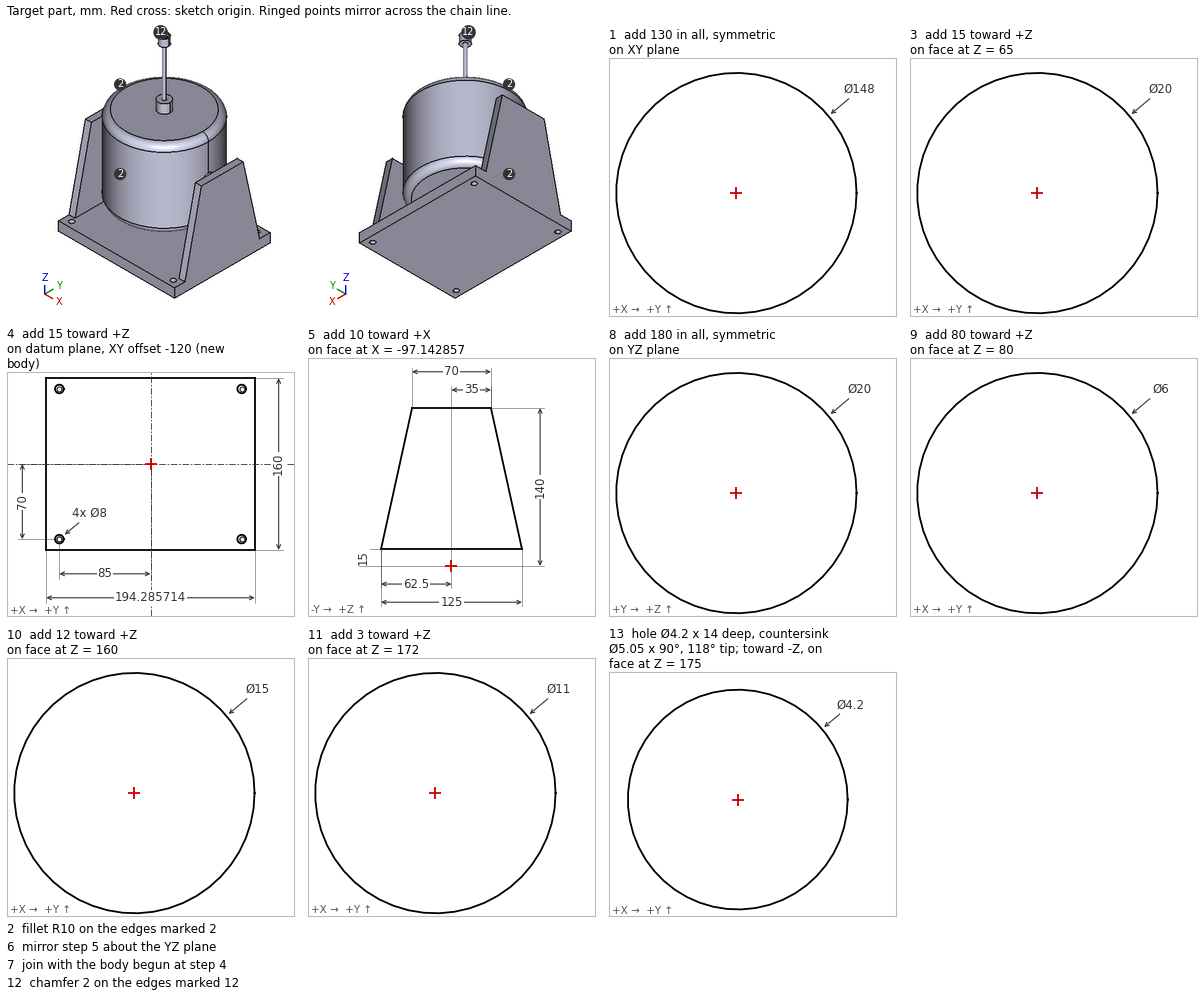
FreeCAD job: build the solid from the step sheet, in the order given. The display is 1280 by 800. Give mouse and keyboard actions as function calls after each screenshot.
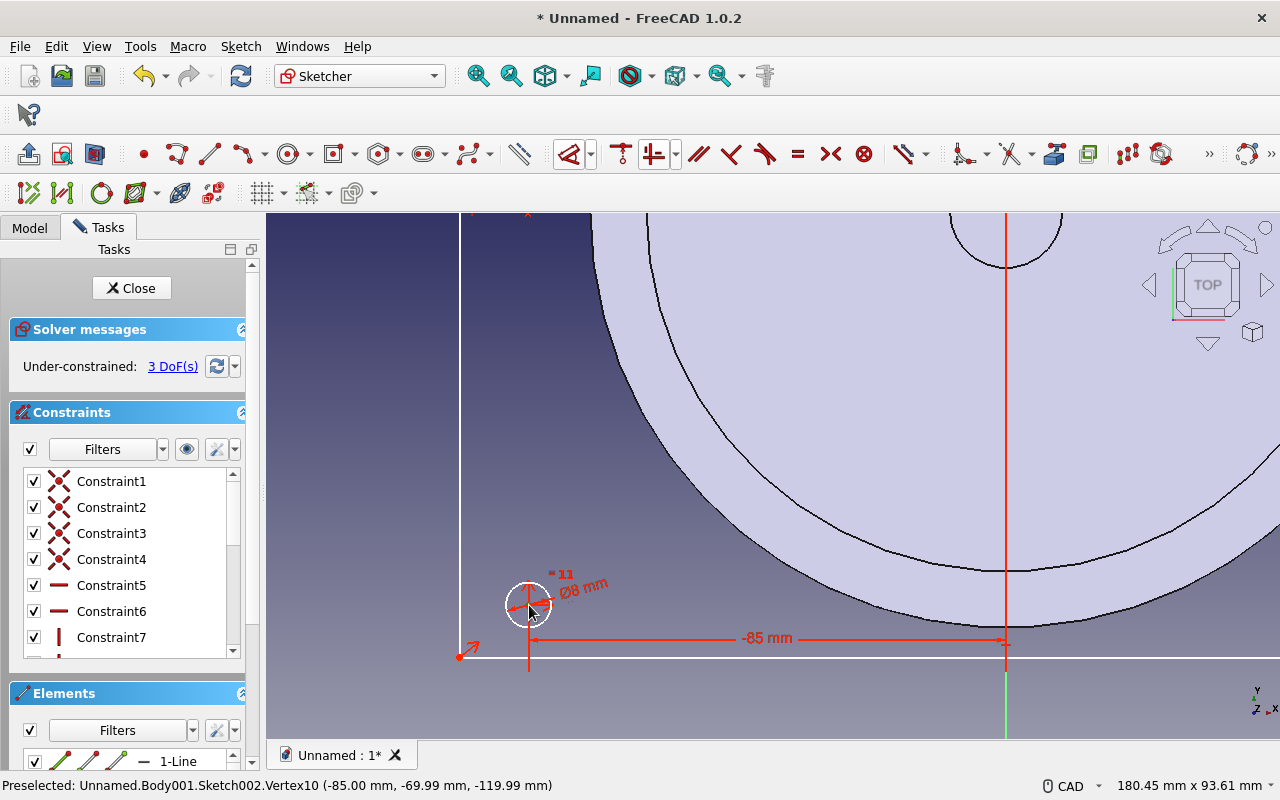
key(i)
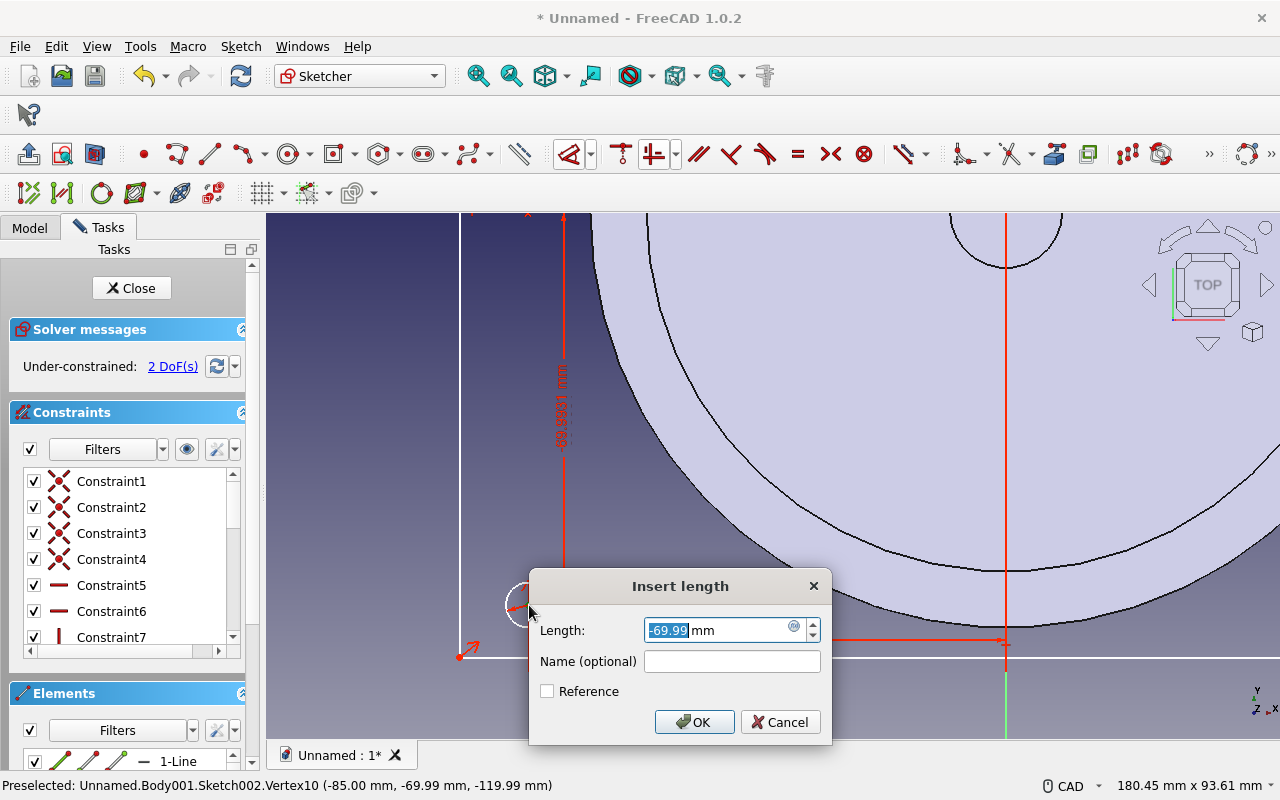
text(-70)
key(Return)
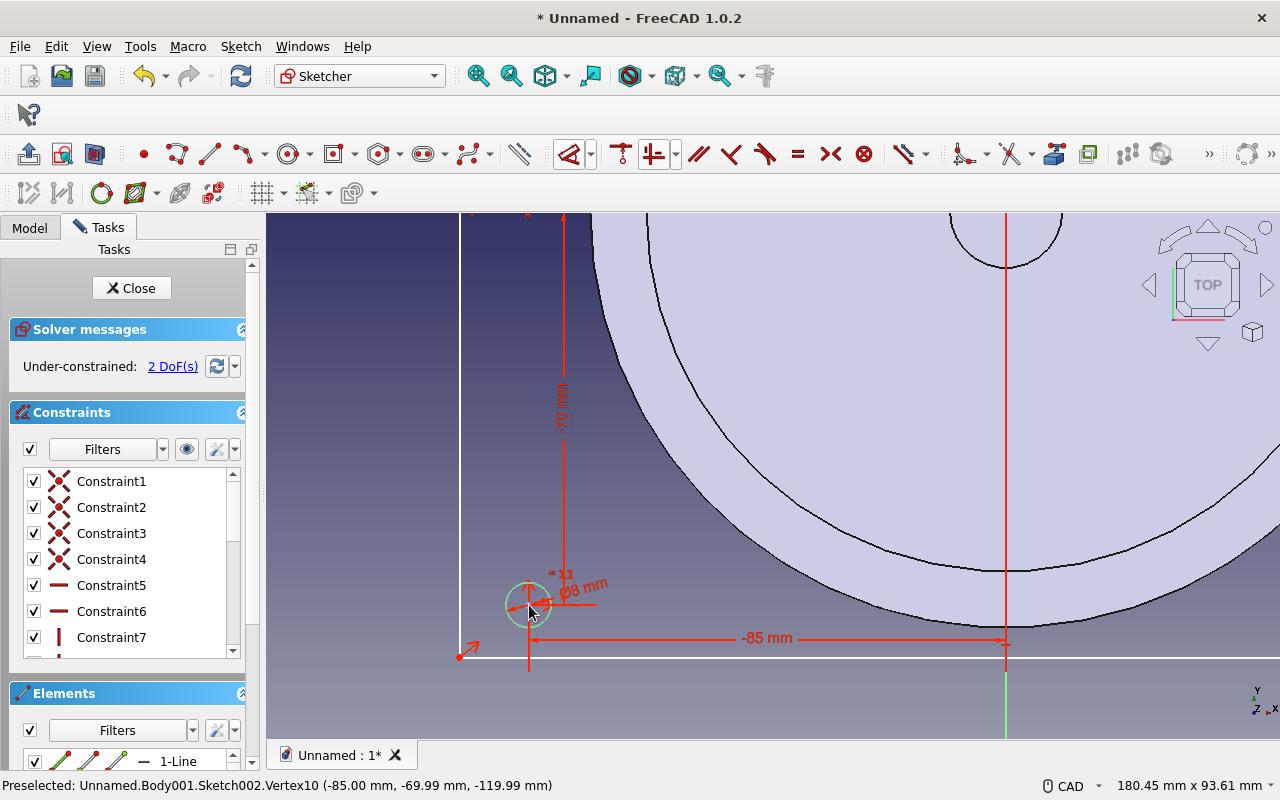
scroll(529, 630, down, 5)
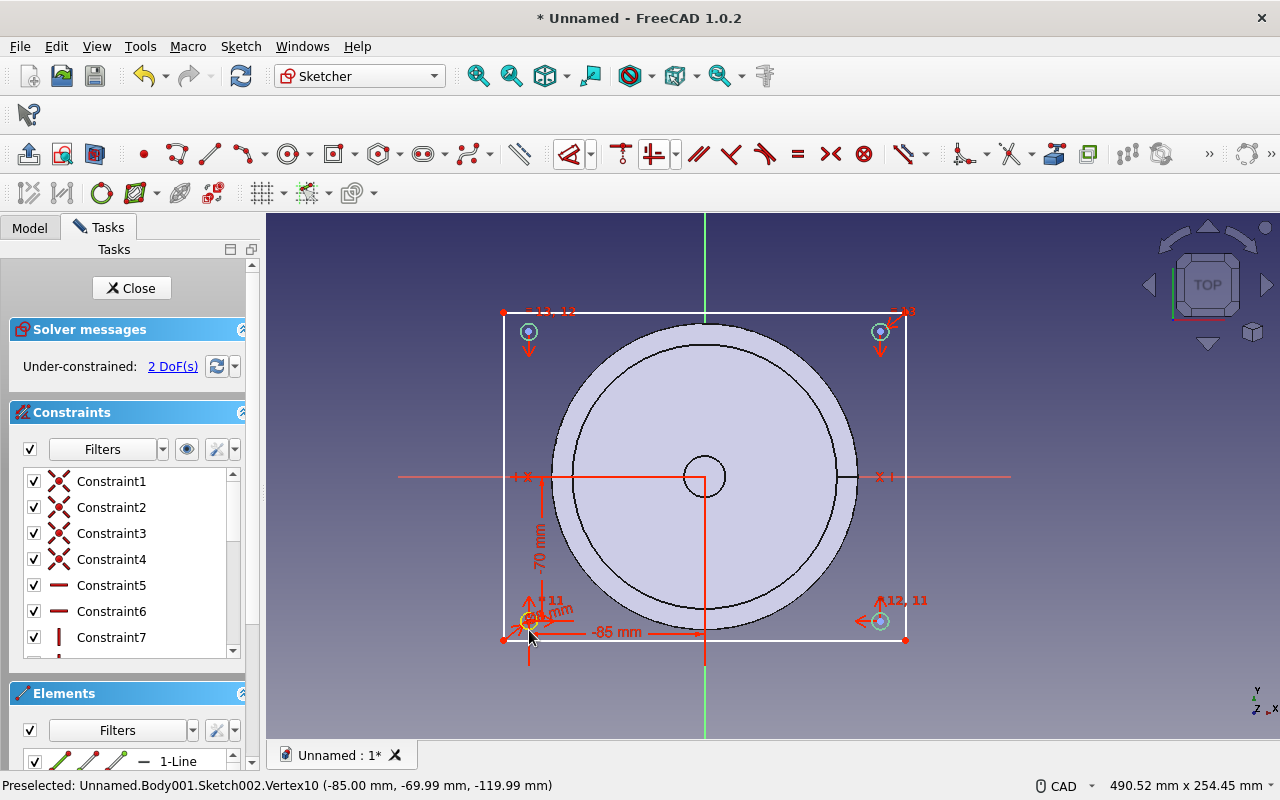
click(906, 542)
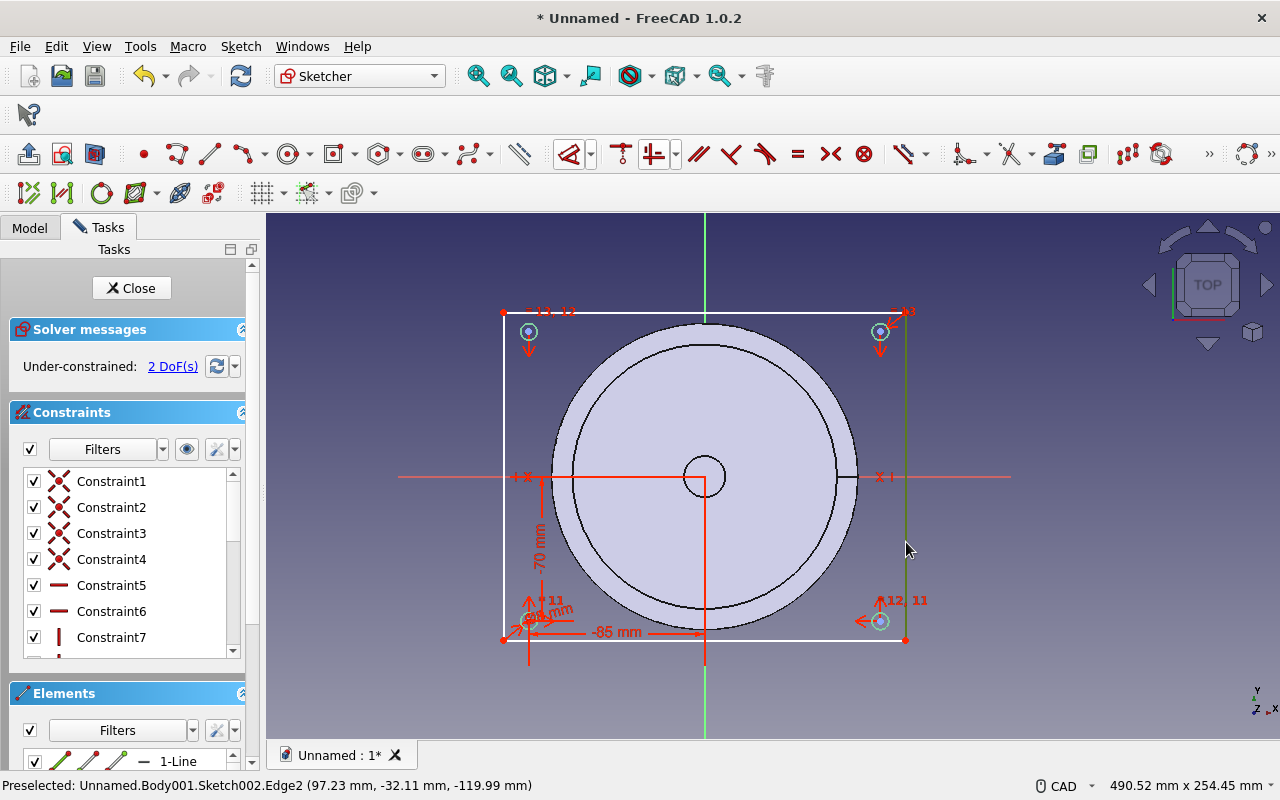
key(i)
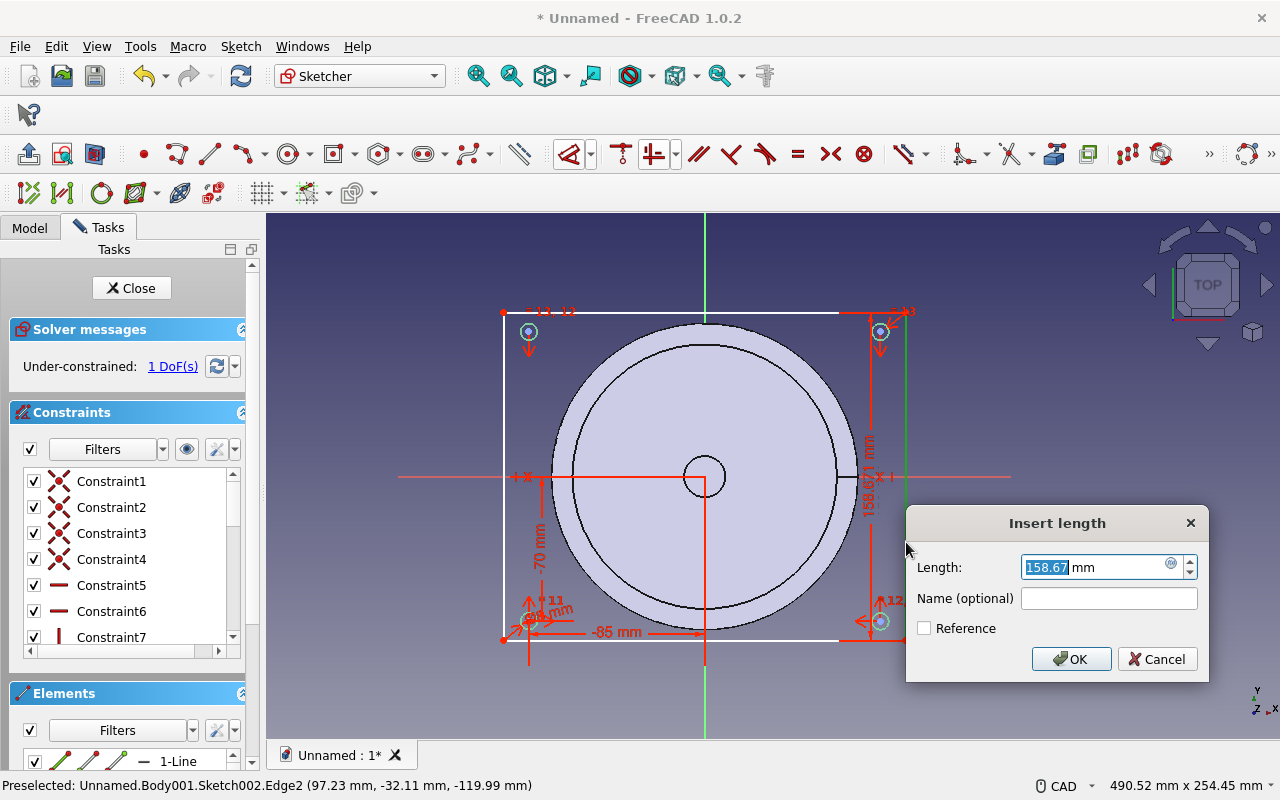
text(160)
key(Return)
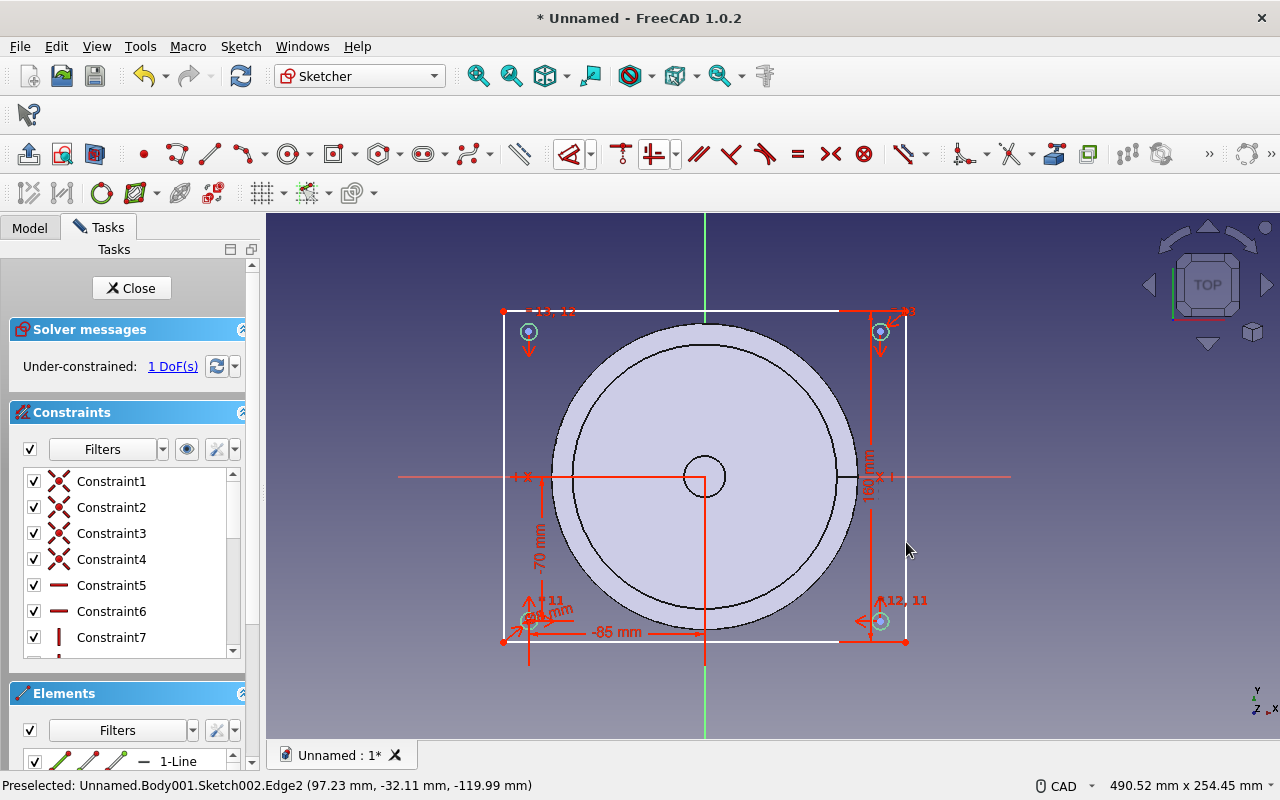
click(624, 642)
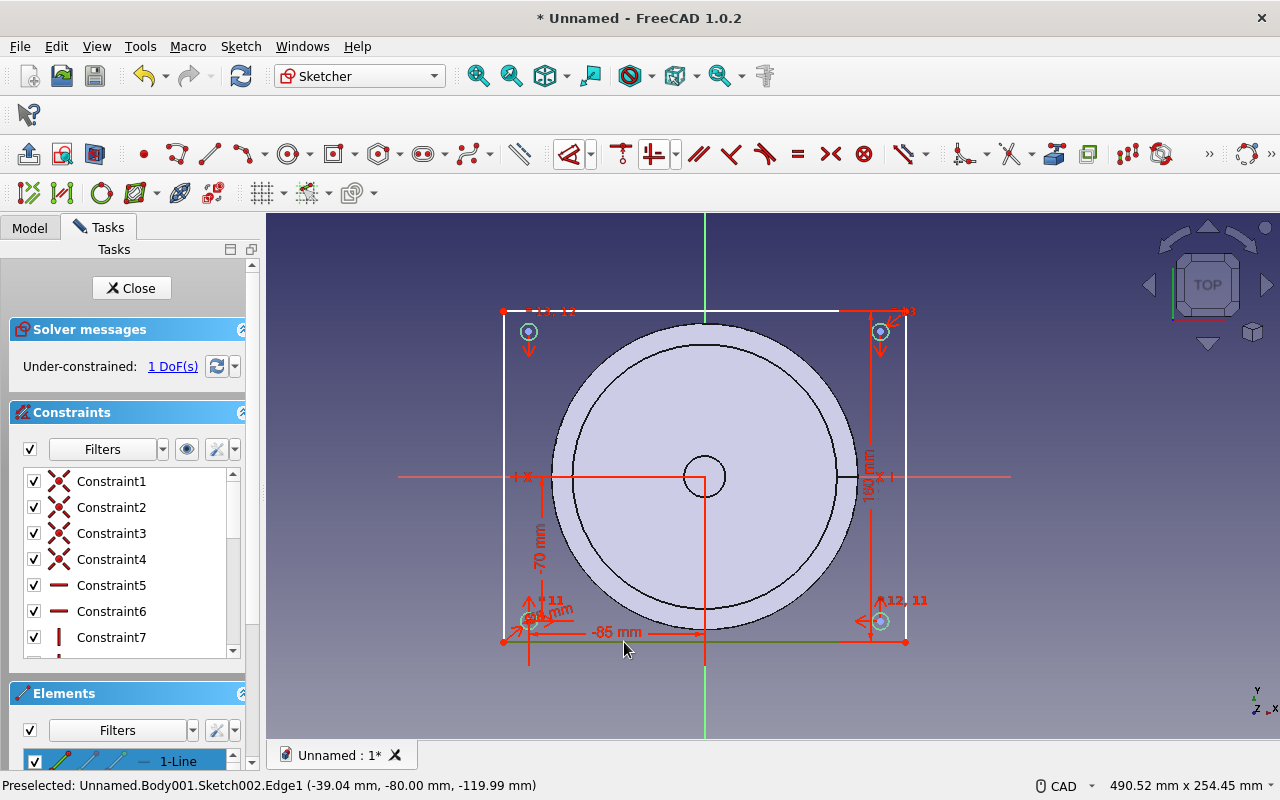
key(l)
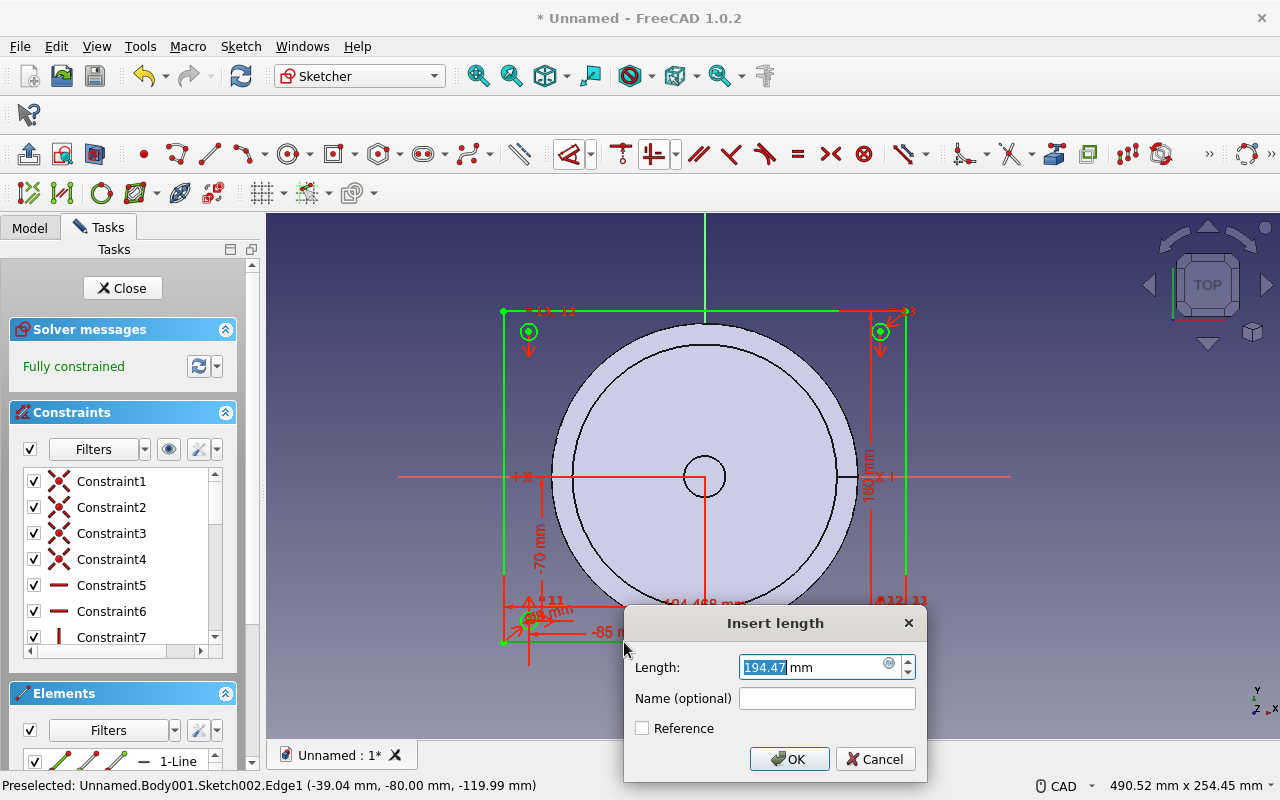
text(194.285714)
key(Return)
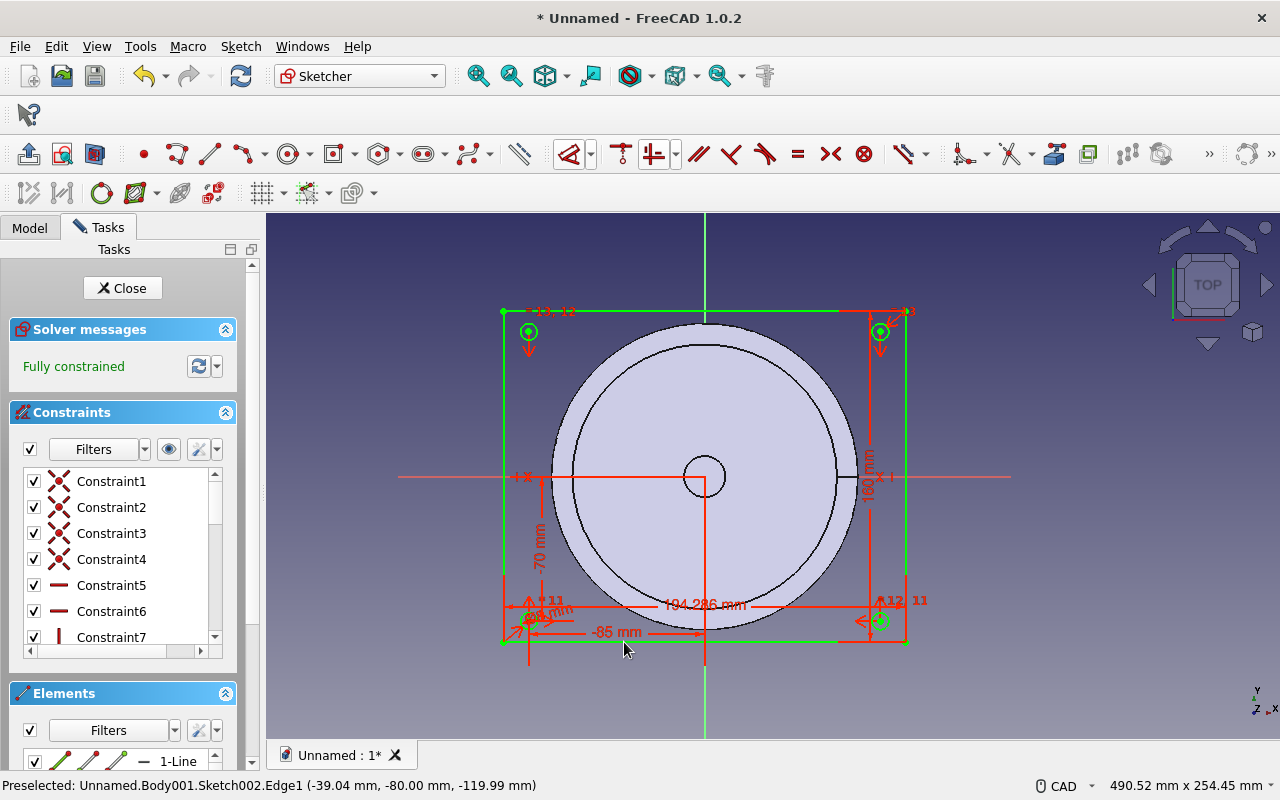
click(123, 288)